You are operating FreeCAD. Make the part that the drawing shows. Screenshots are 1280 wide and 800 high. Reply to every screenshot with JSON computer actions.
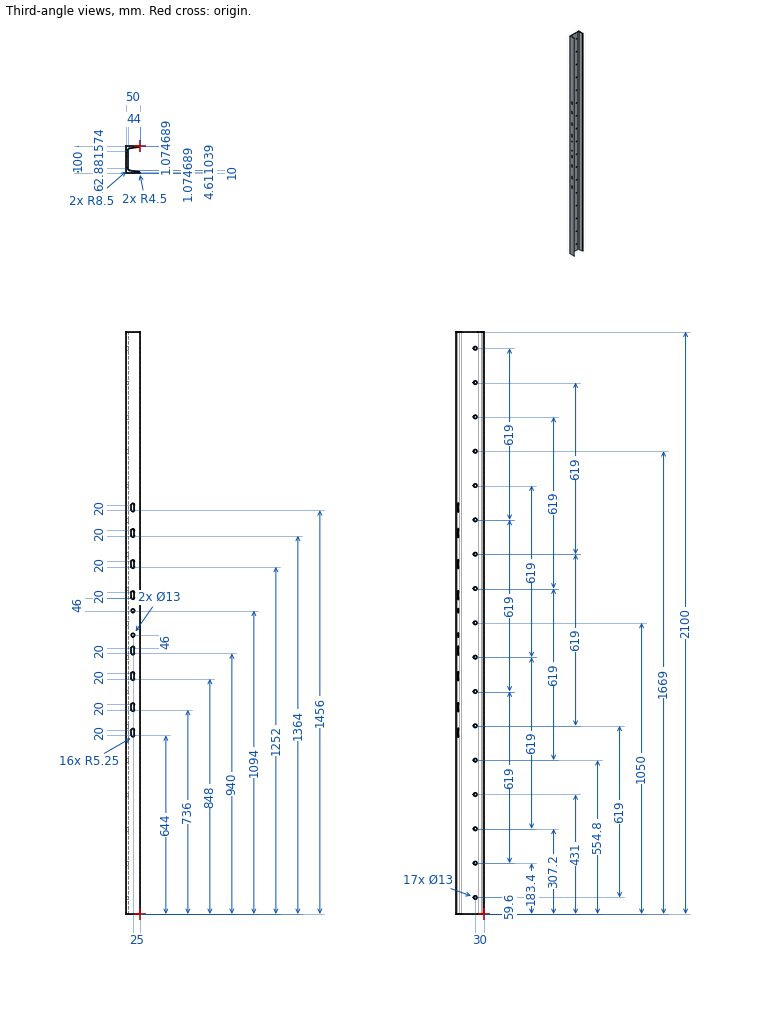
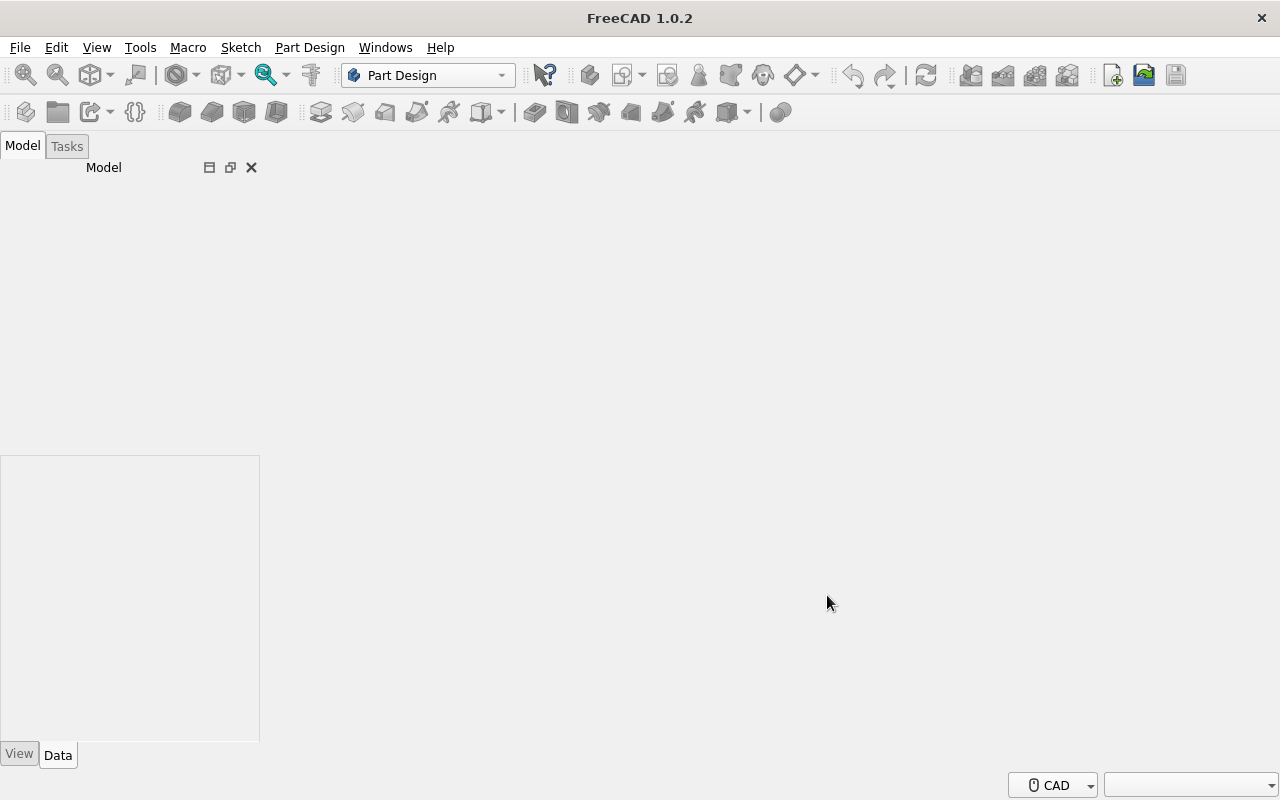
{"action": "key", "text": "ctrl+n"}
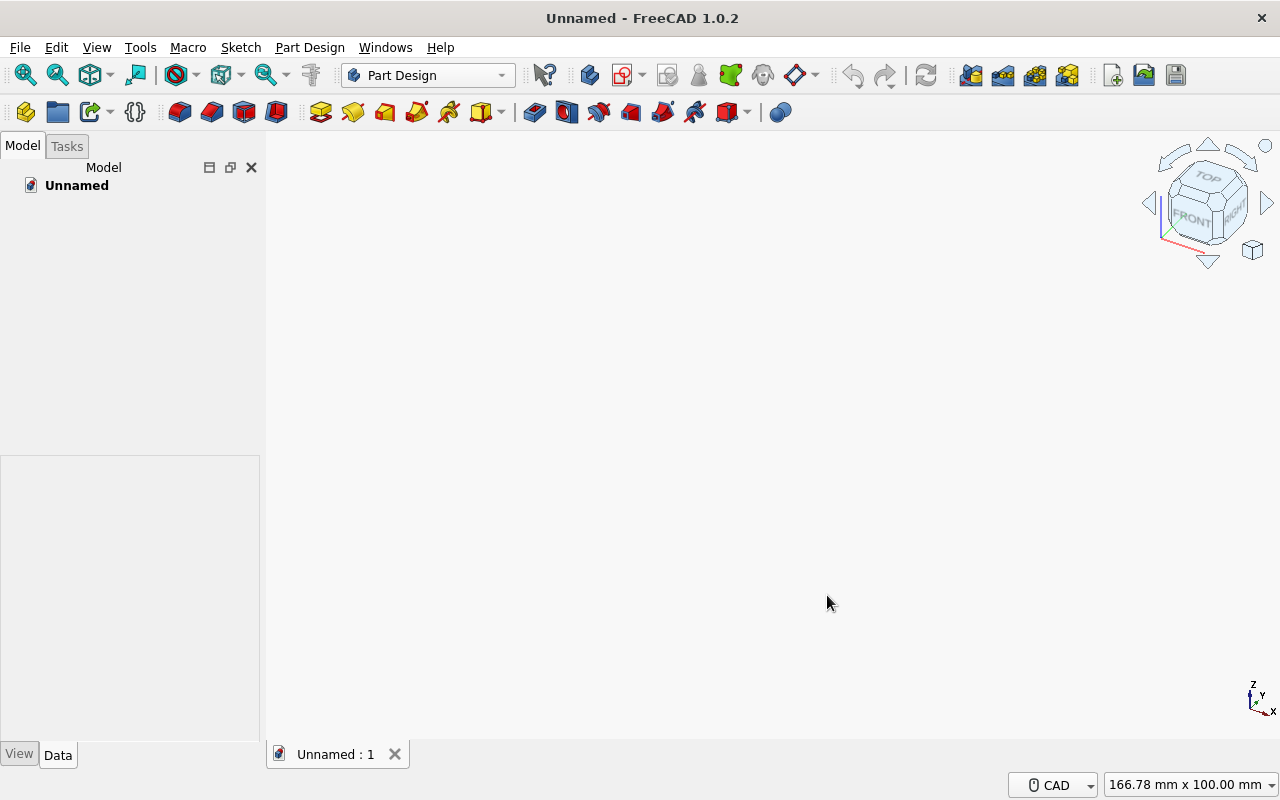
{"action": "left_click", "coordinate": [622, 76]}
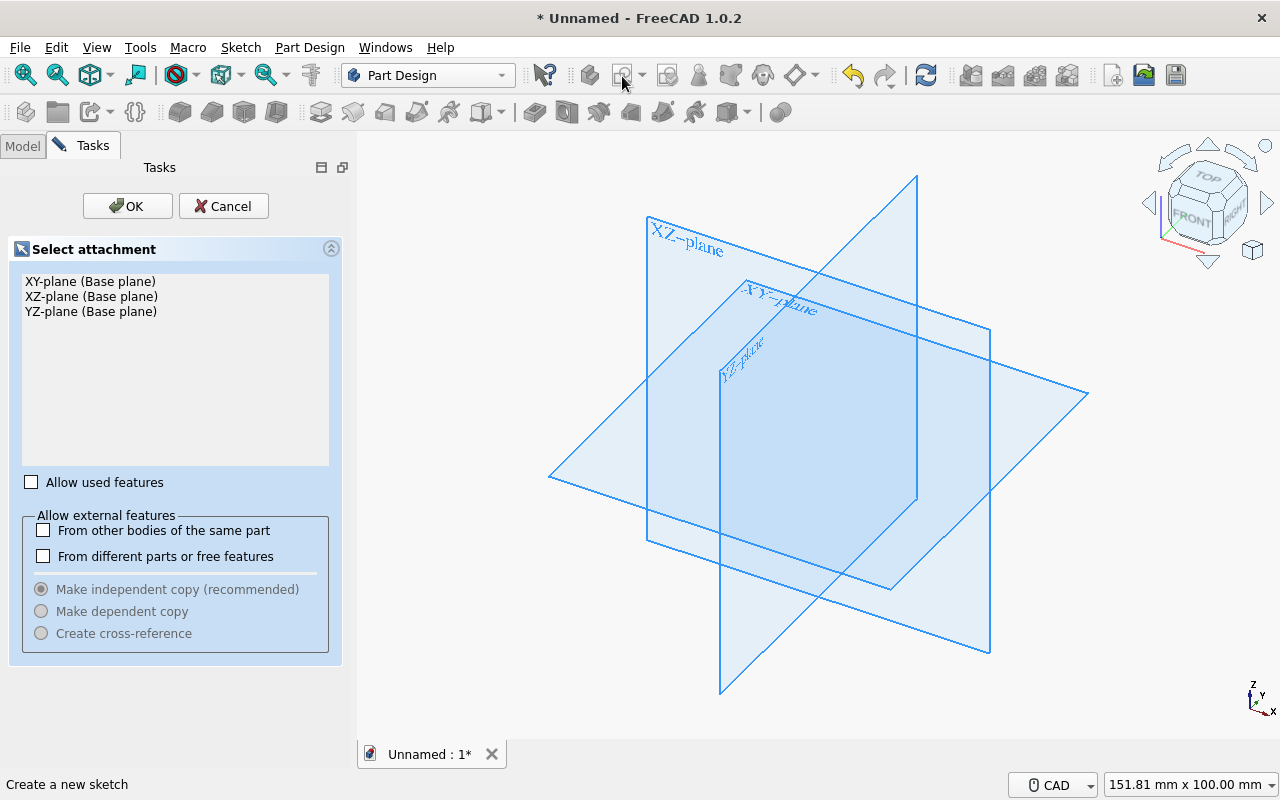
{"action": "left_click", "coordinate": [82, 282]}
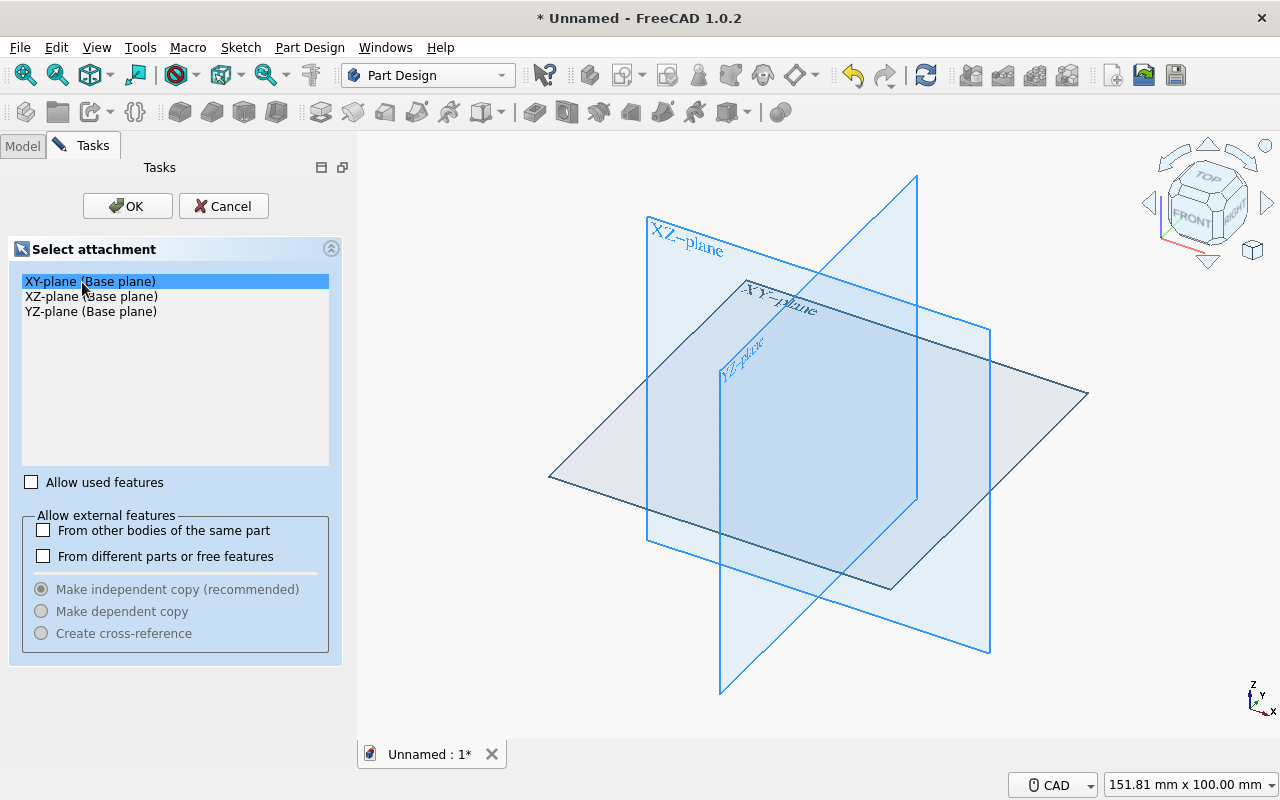
{"action": "left_click", "coordinate": [128, 206]}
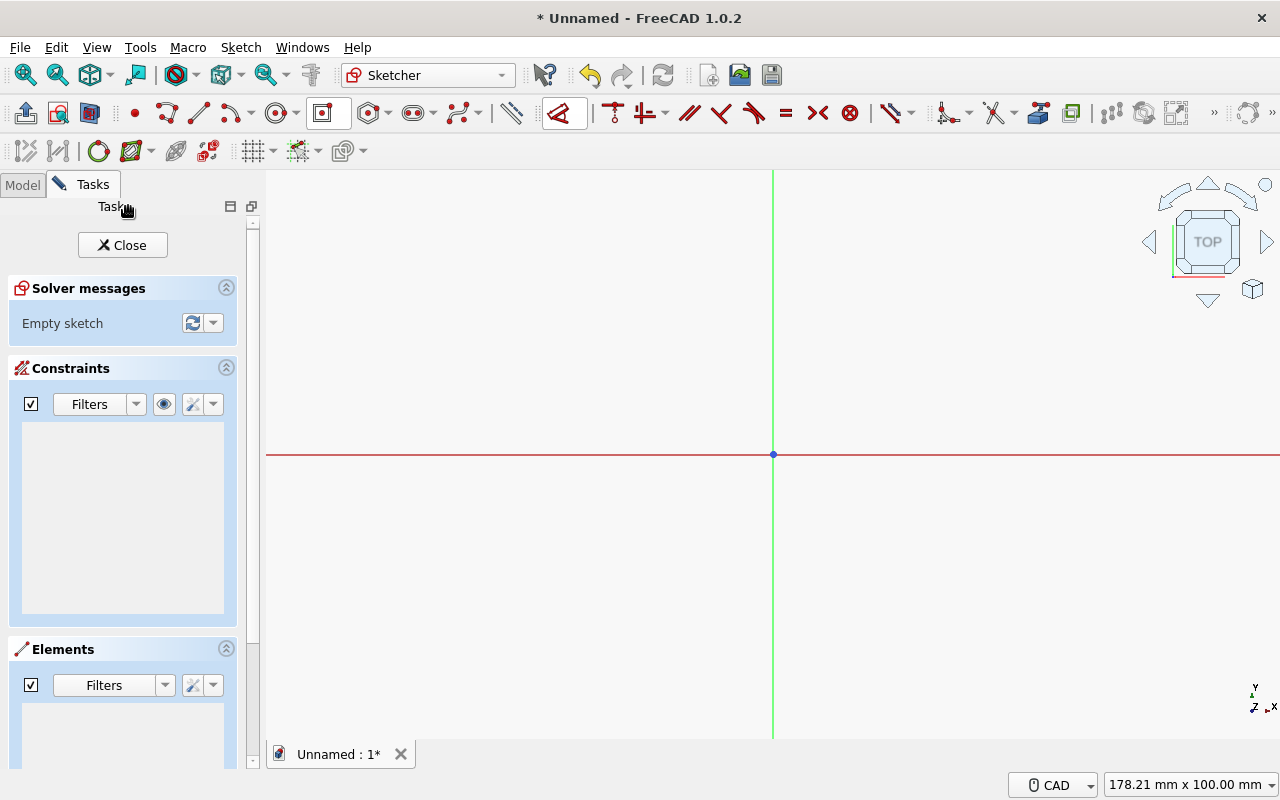
{"action": "scroll", "coordinate": [794, 198], "scroll_direction": "down", "scroll_amount": 3}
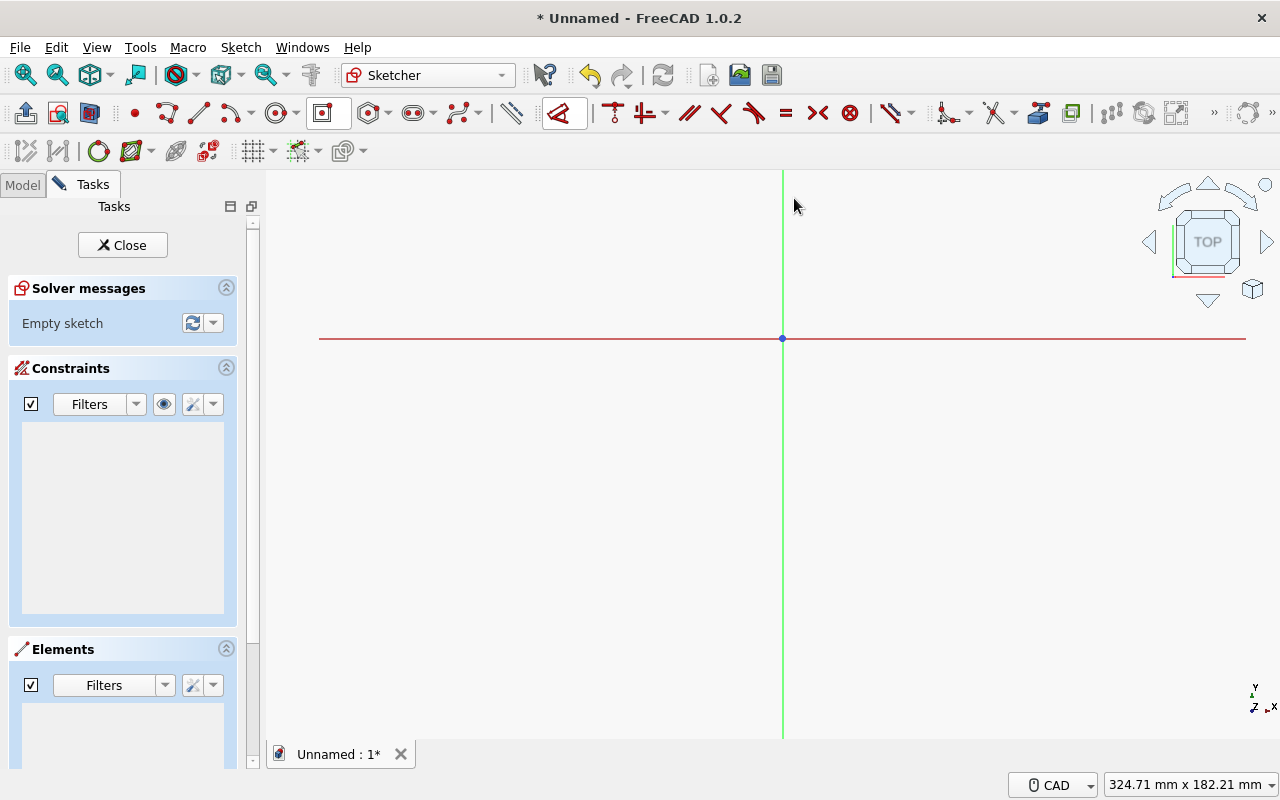
{"action": "key", "text": "g l"}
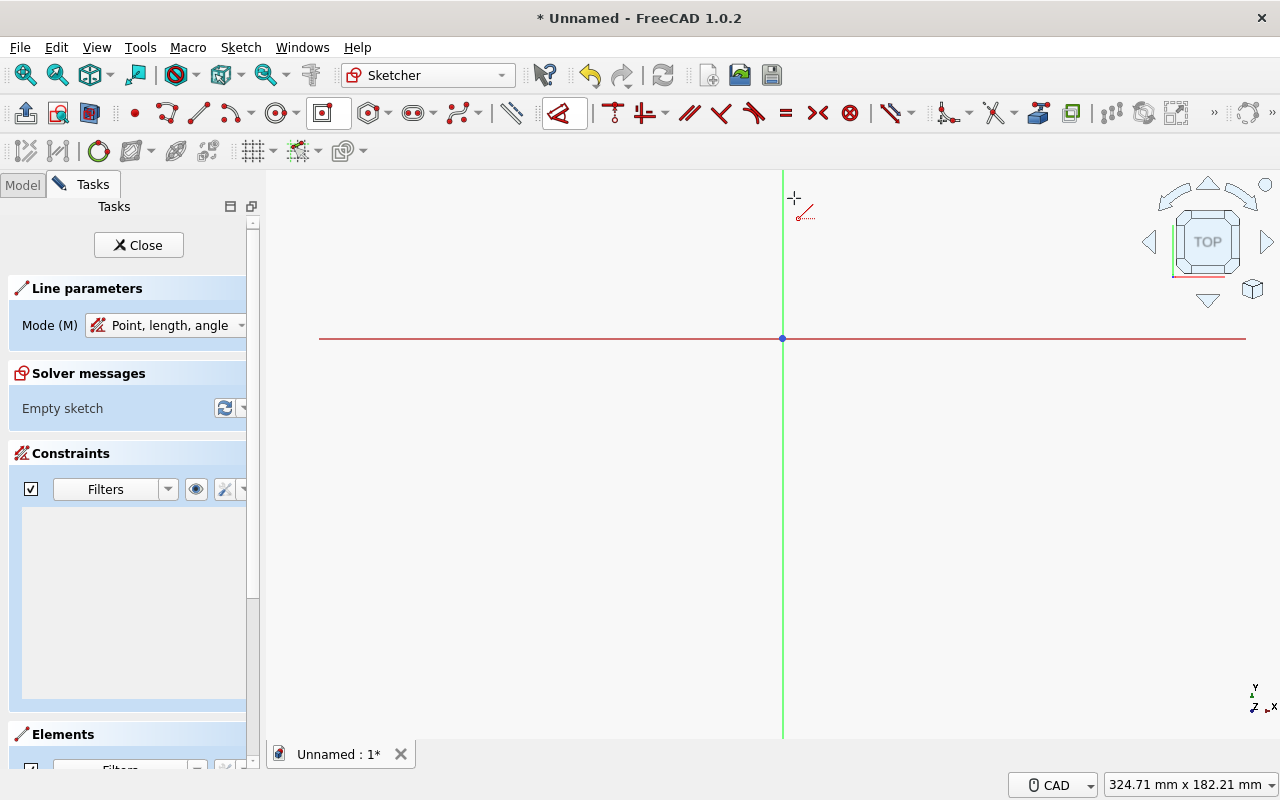
{"action": "scroll", "coordinate": [771, 634], "scroll_direction": "up", "scroll_amount": 2}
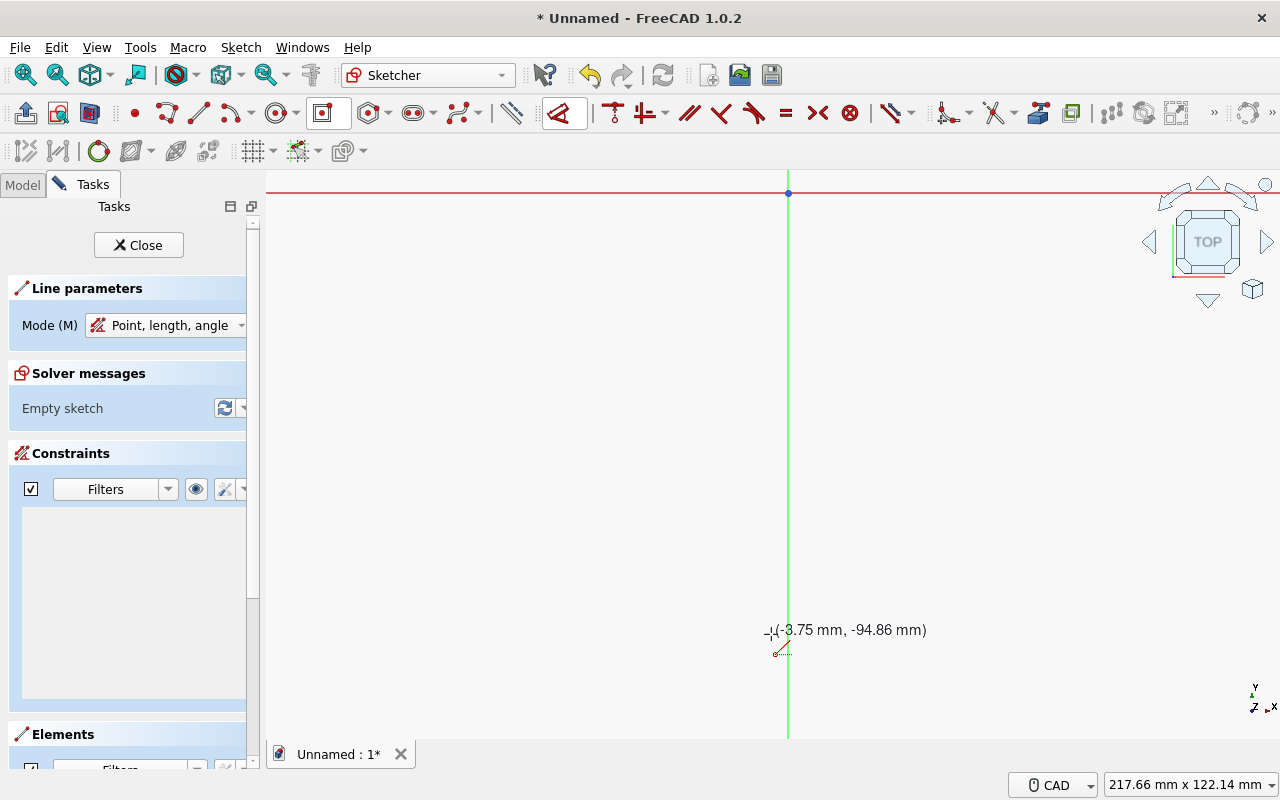
{"action": "left_click", "coordinate": [770, 633]}
{"action": "left_click", "coordinate": [617, 612]}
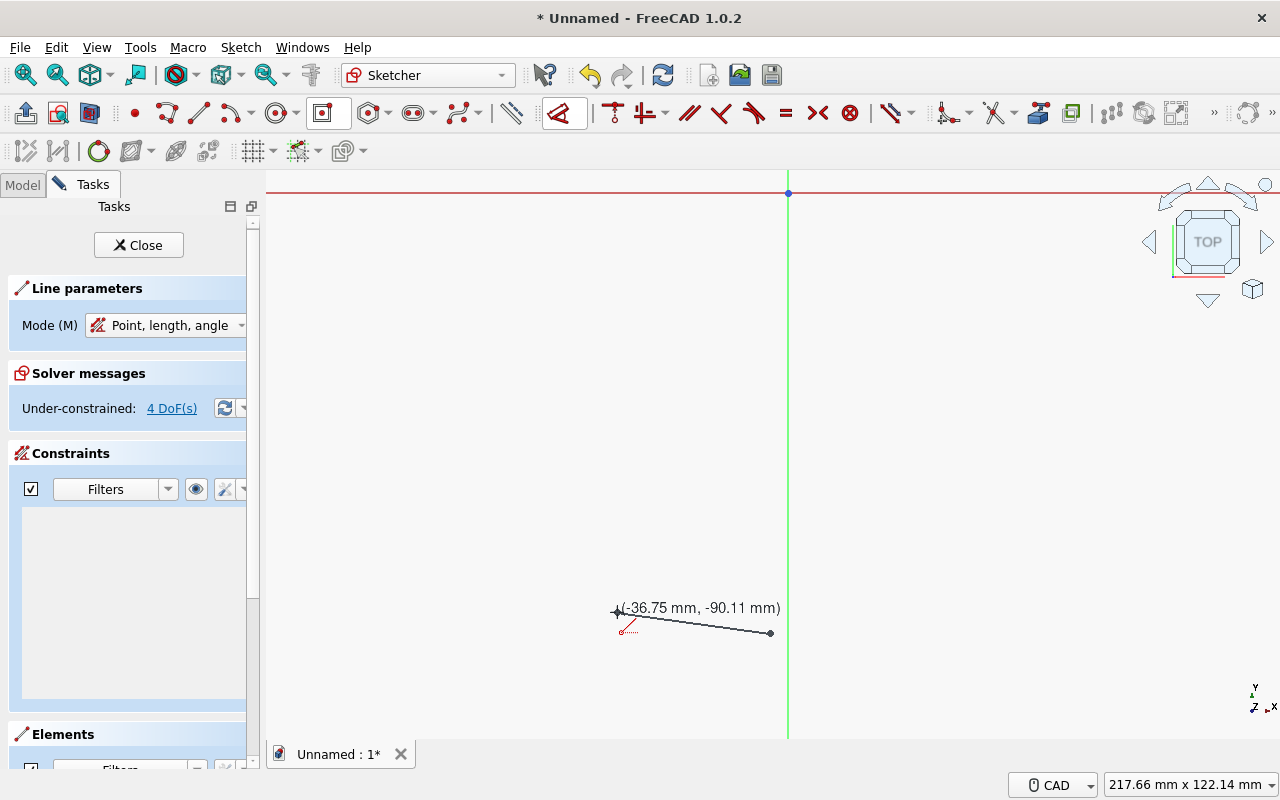
{"action": "left_click", "coordinate": [583, 573]}
{"action": "left_click", "coordinate": [583, 280]}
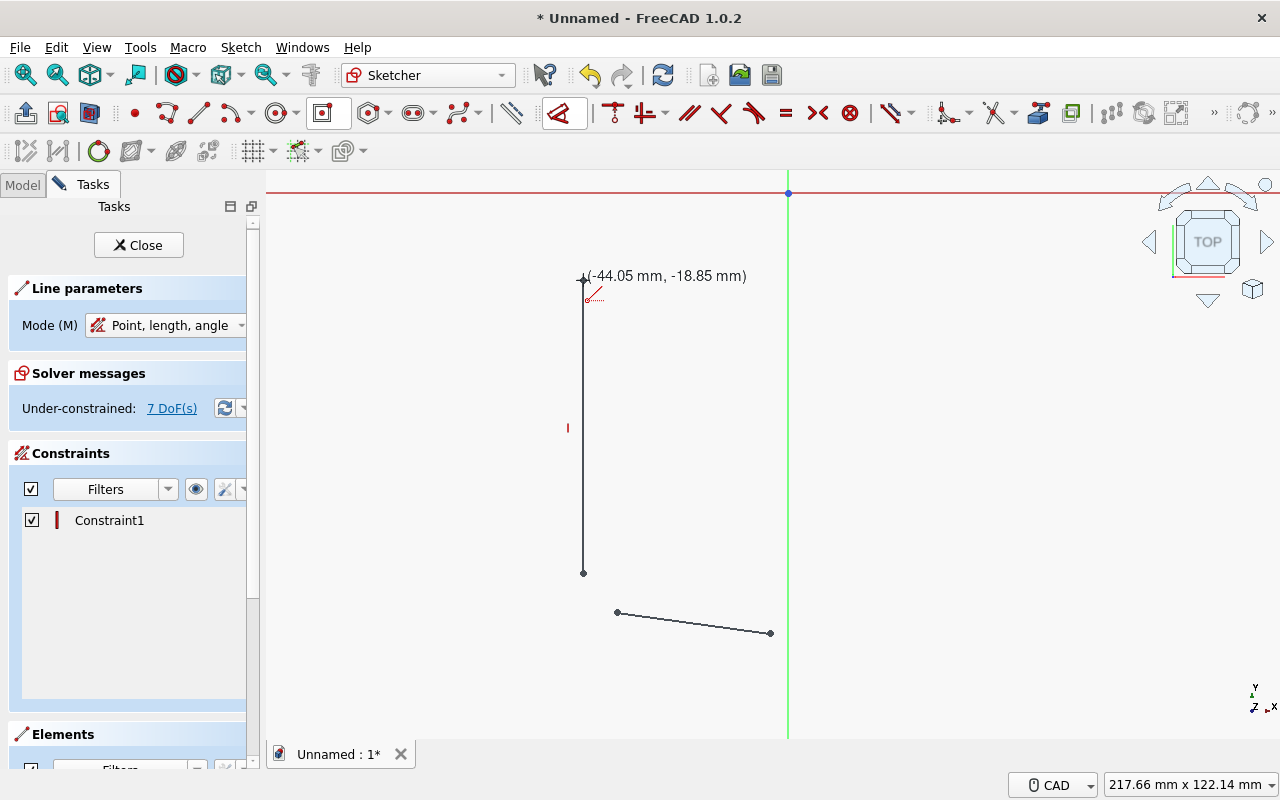
{"action": "left_click", "coordinate": [617, 240]}
{"action": "left_click", "coordinate": [770, 219]}